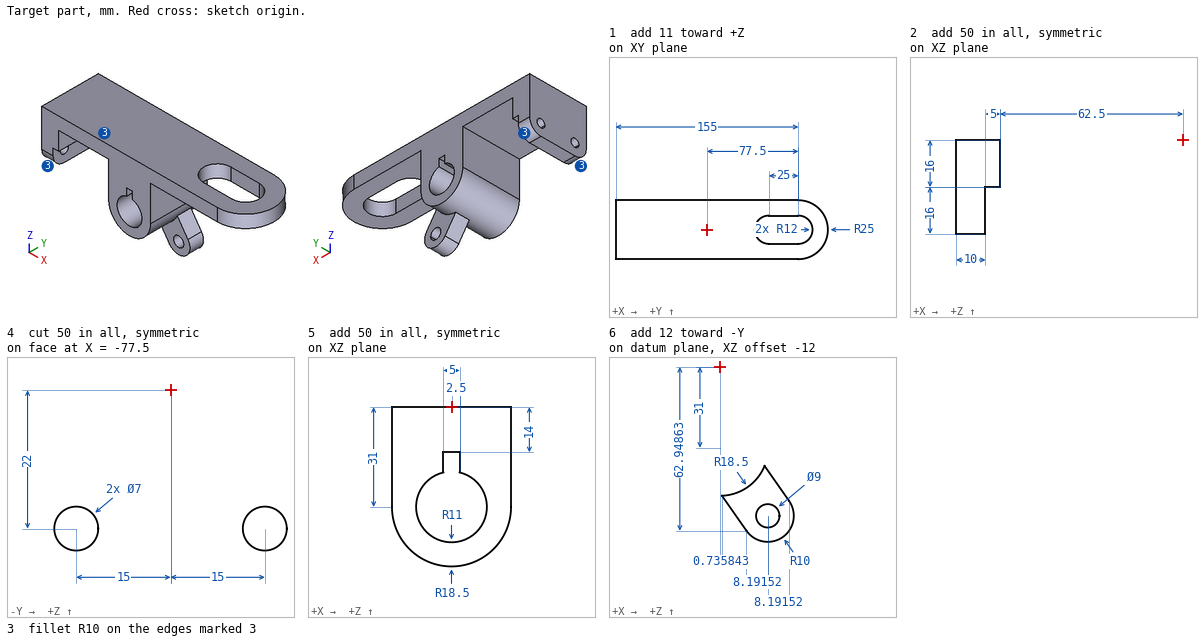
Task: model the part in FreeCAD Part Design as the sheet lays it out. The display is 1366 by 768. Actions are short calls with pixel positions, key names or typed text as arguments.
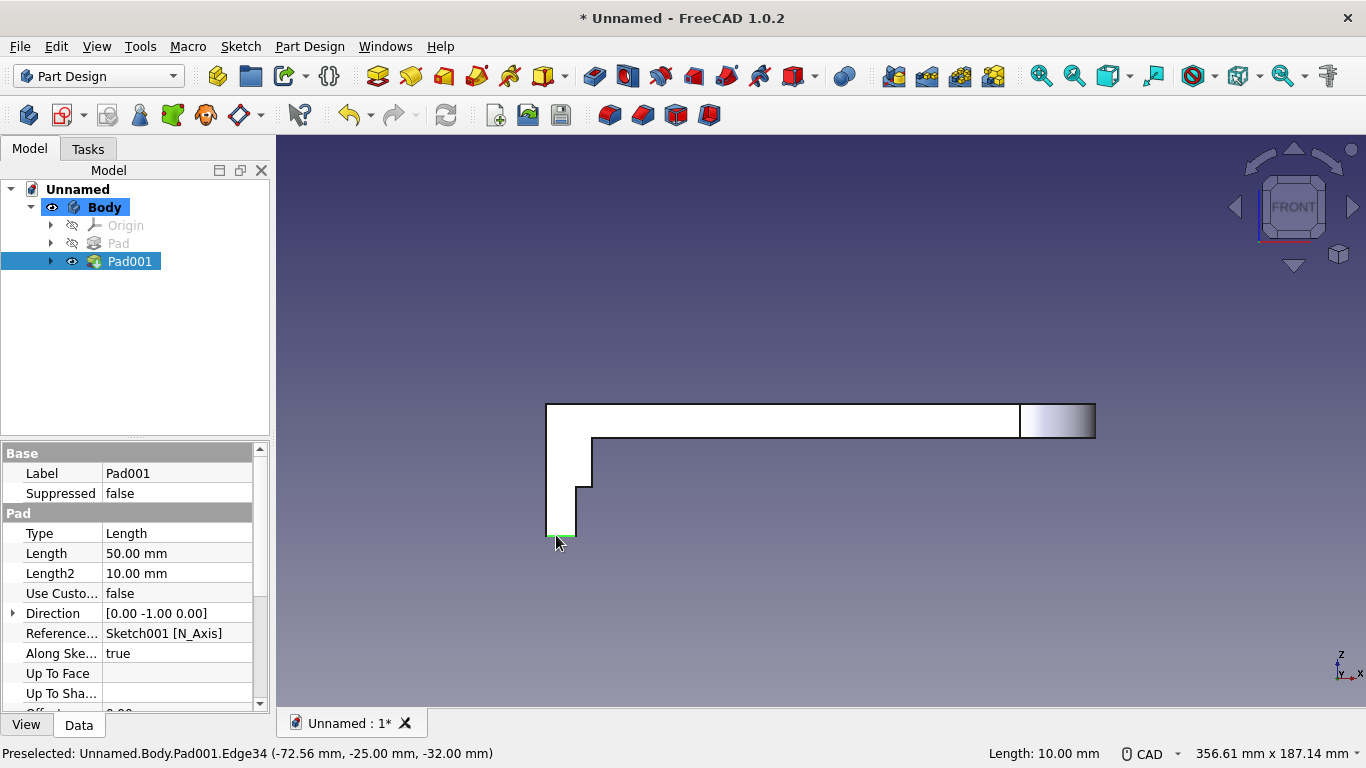
key(3)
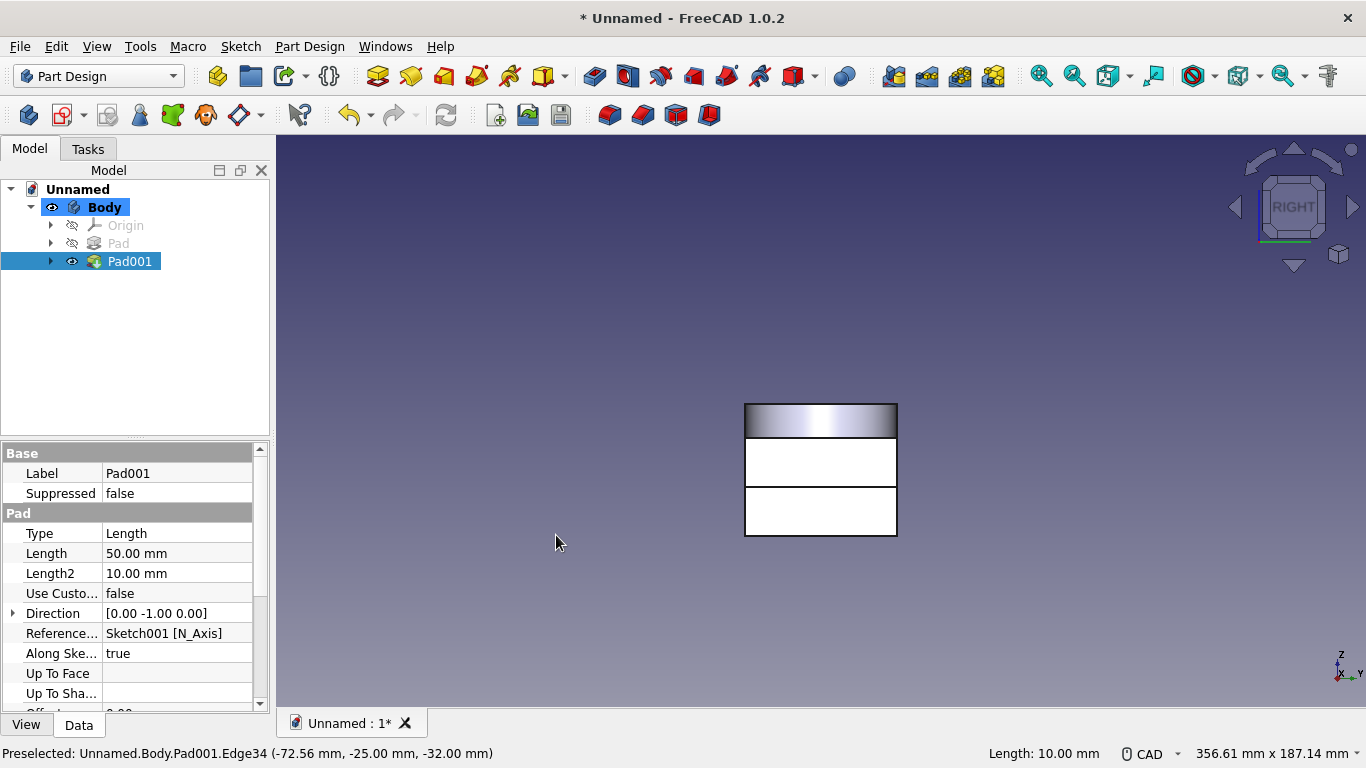
key(v)
key(f)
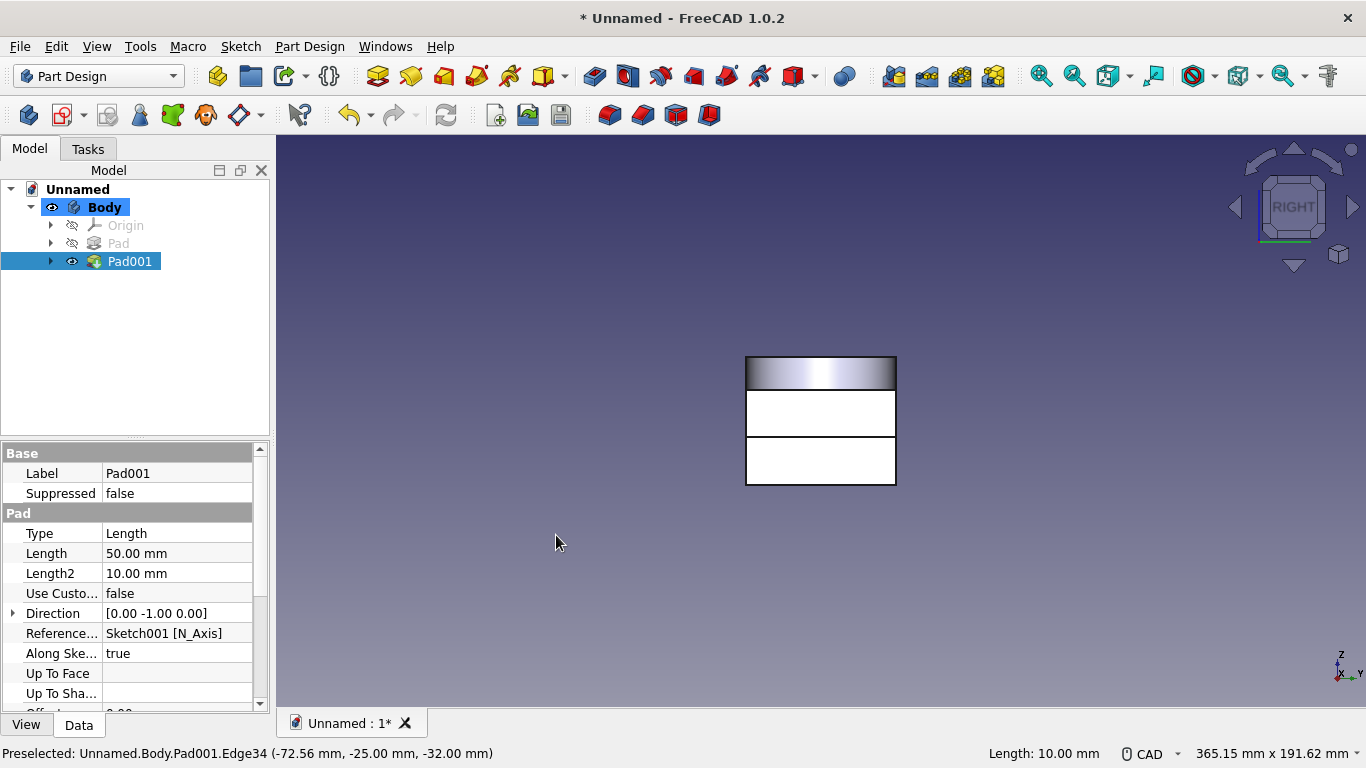
key(5)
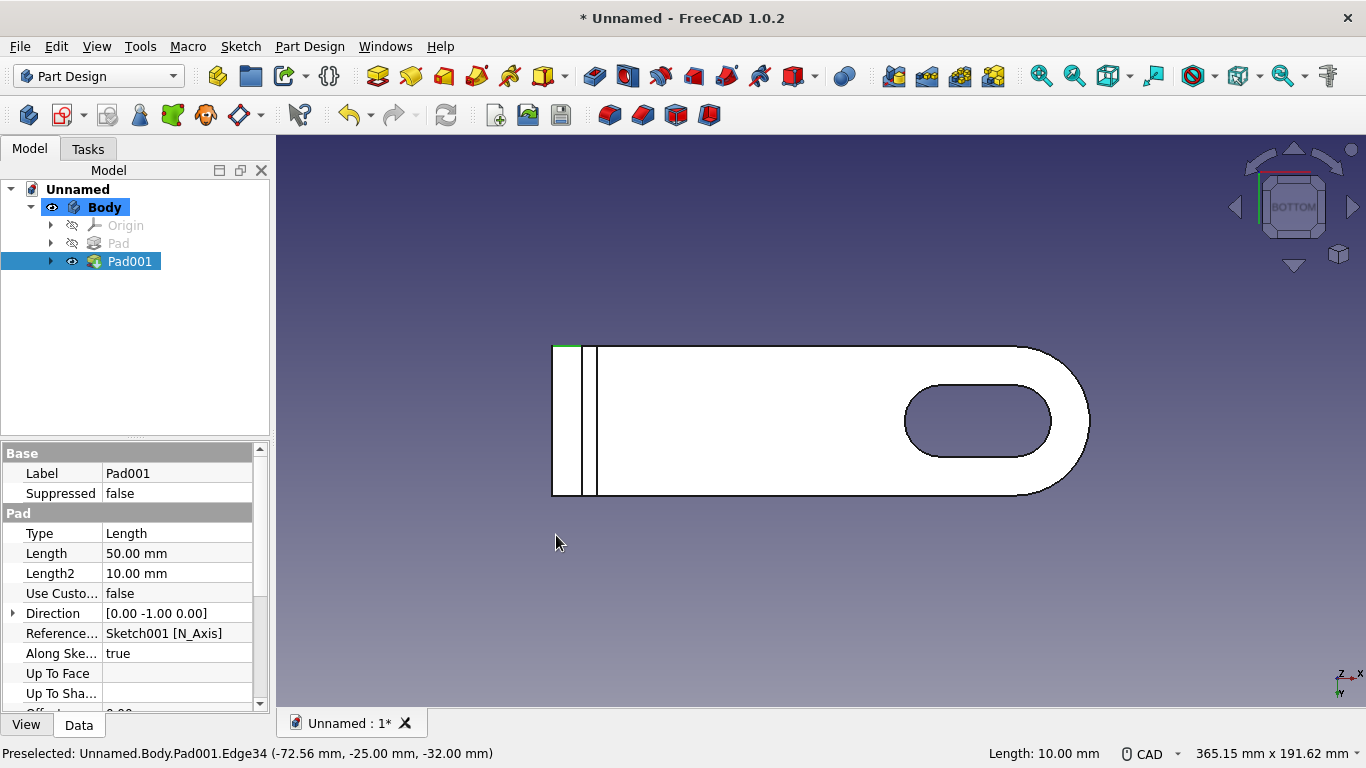
click(567, 495, ctrl)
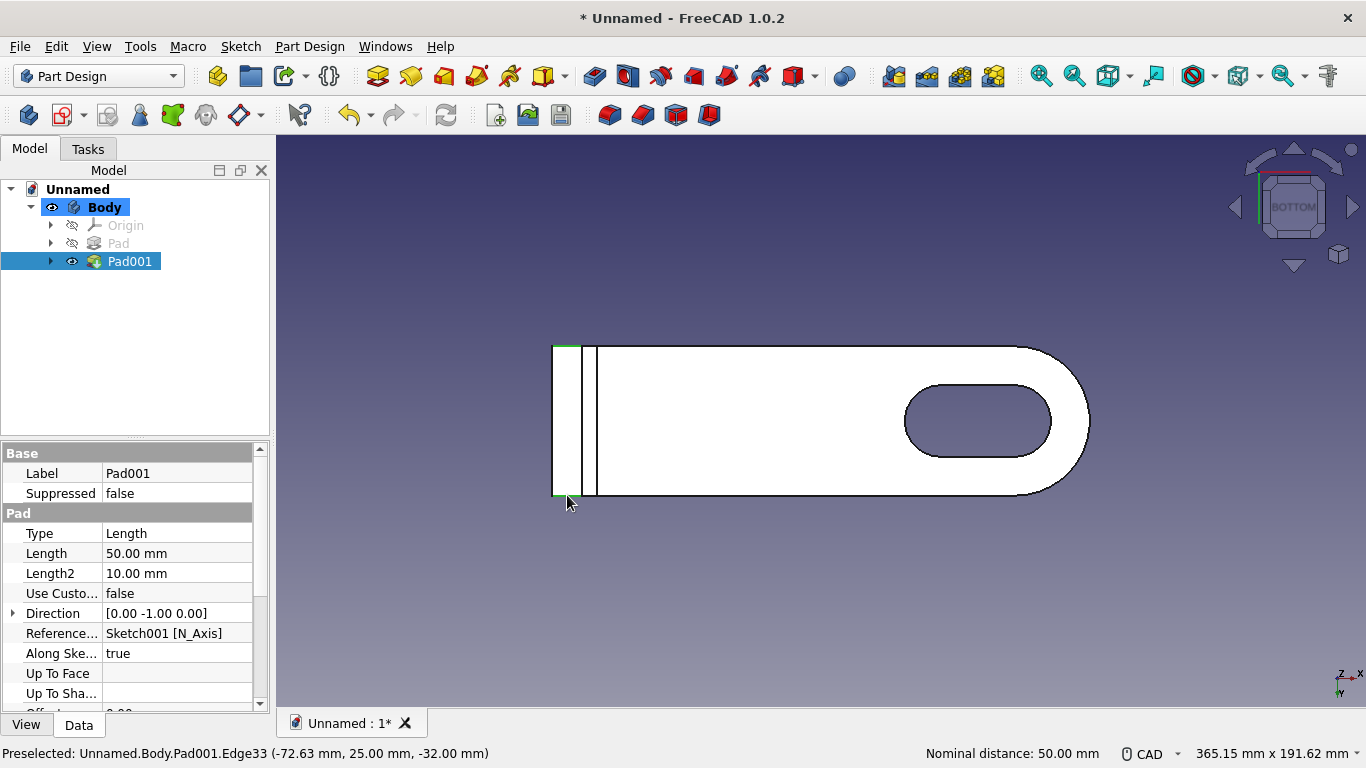
click(610, 116)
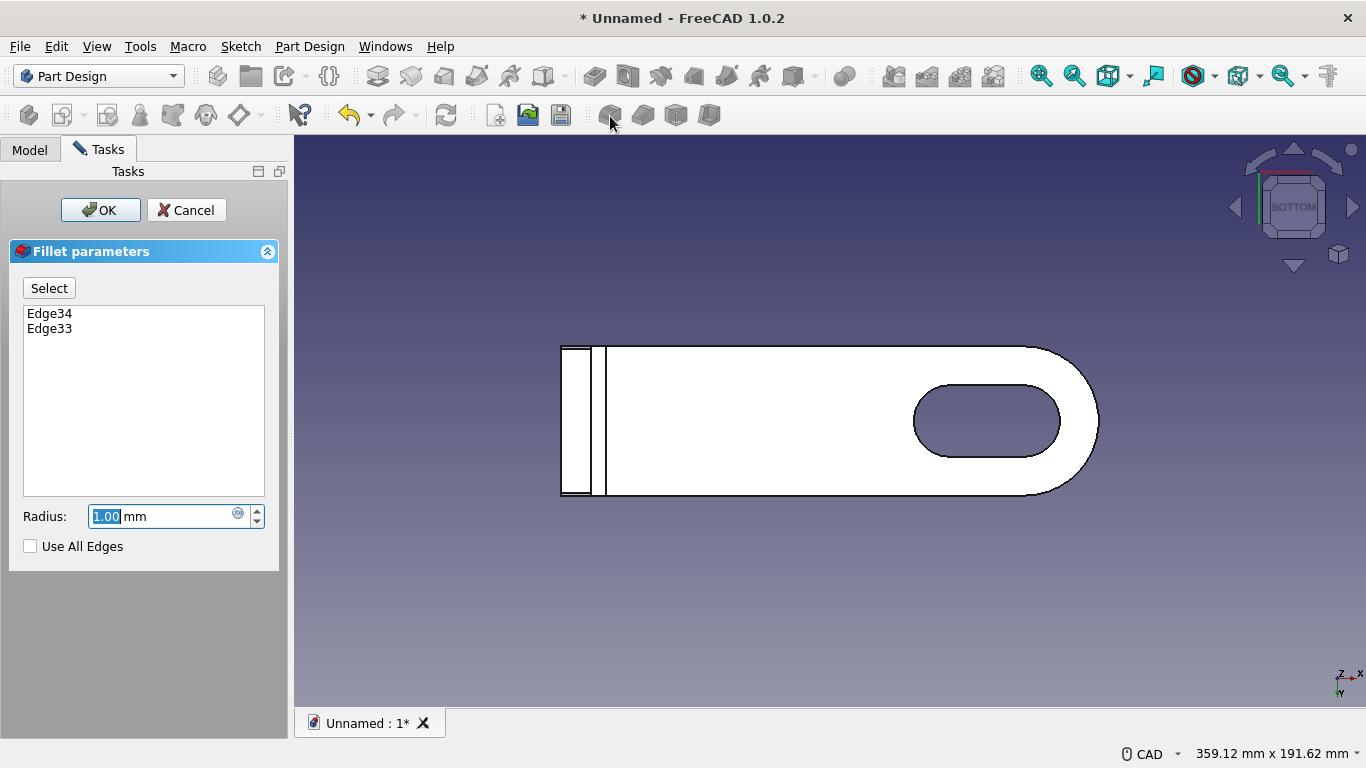
text(10)
key(Tab)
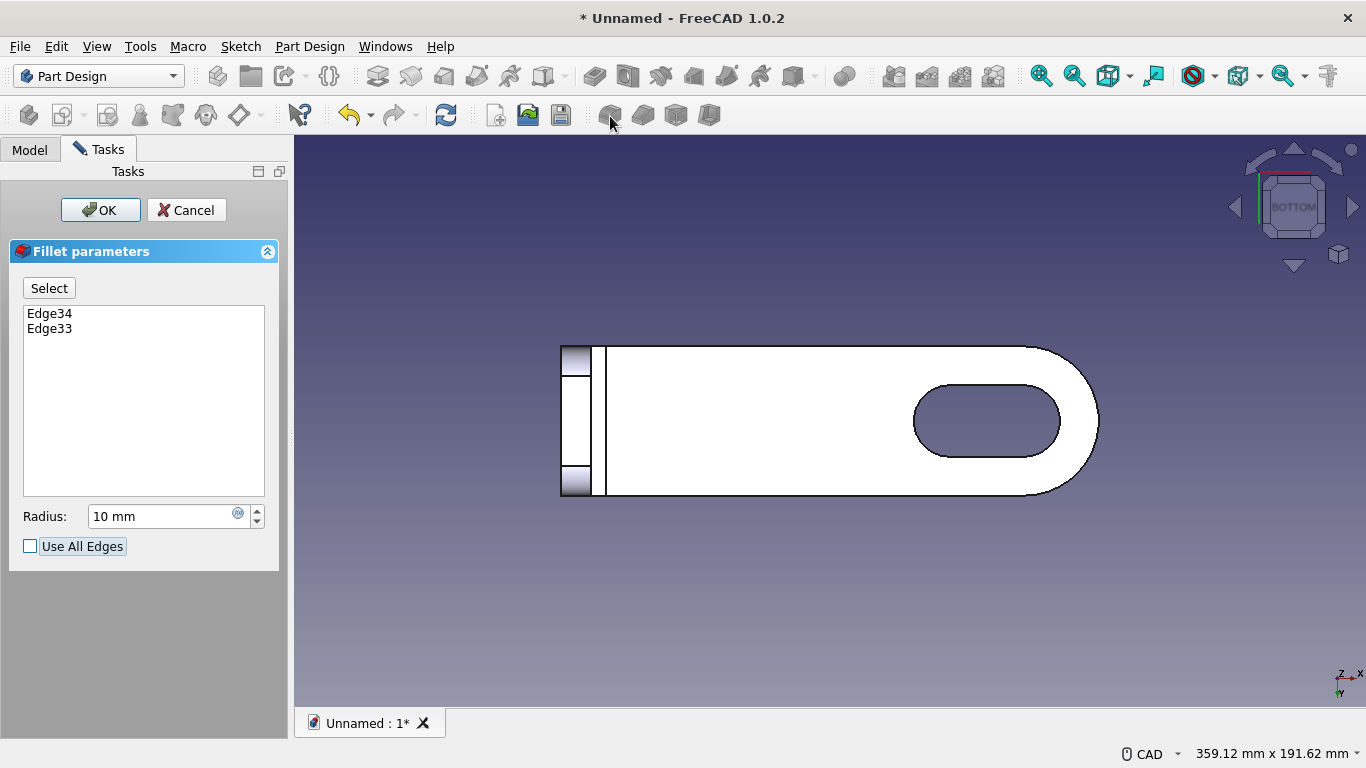
click(101, 210)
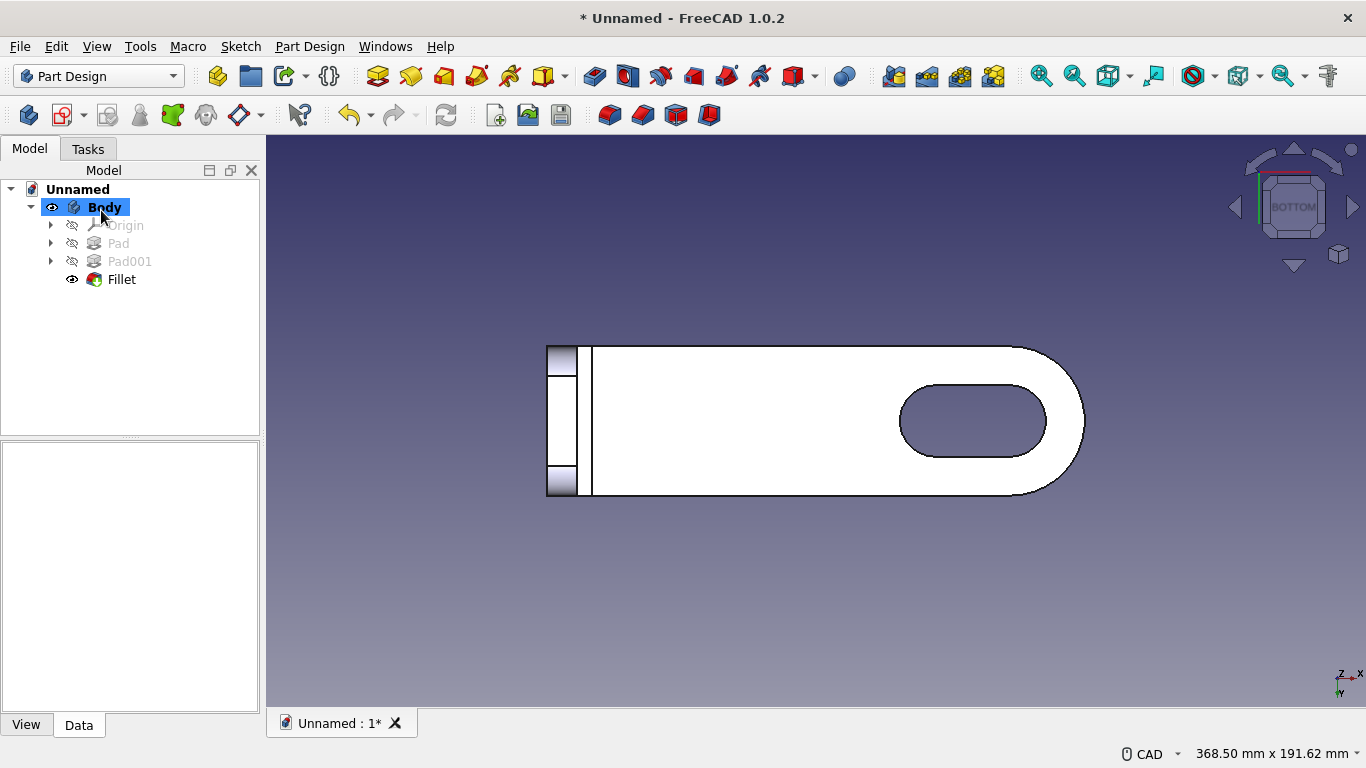
key(6)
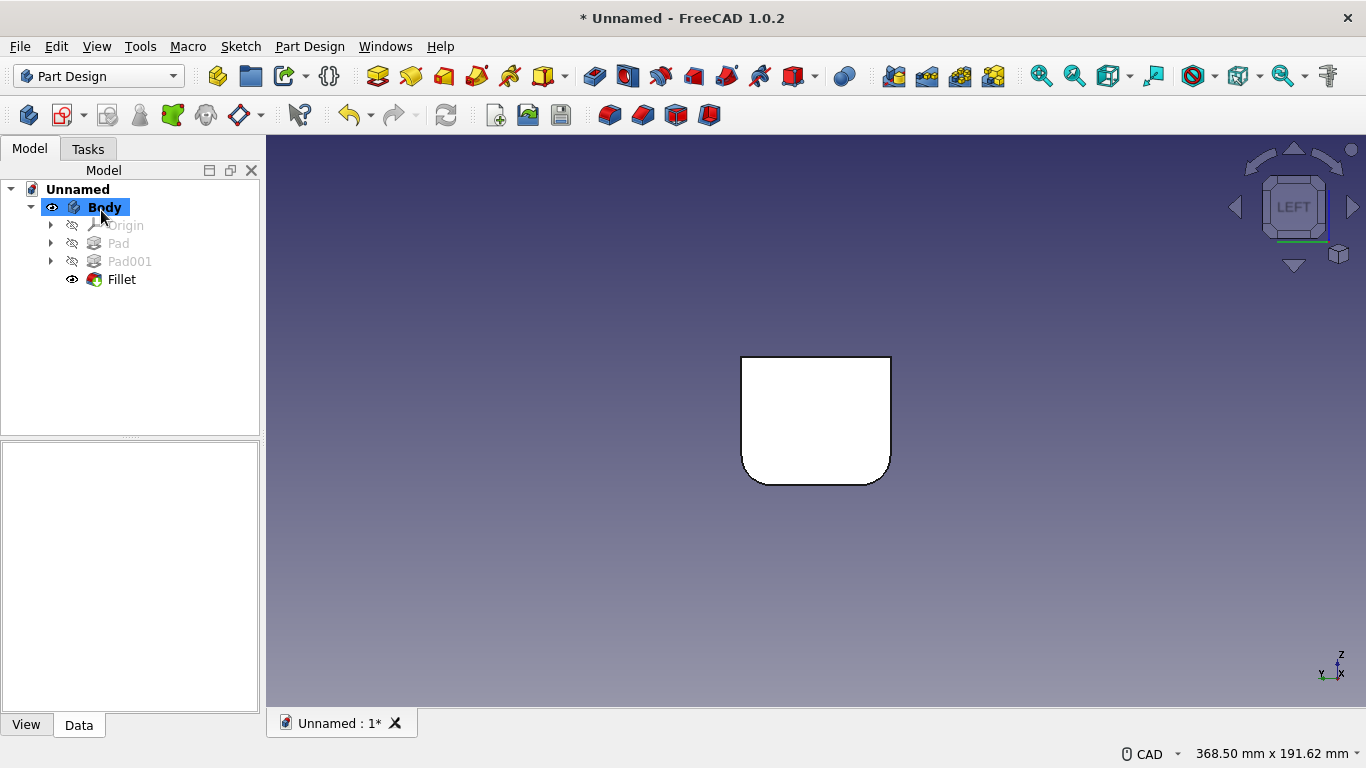
click(1042, 76)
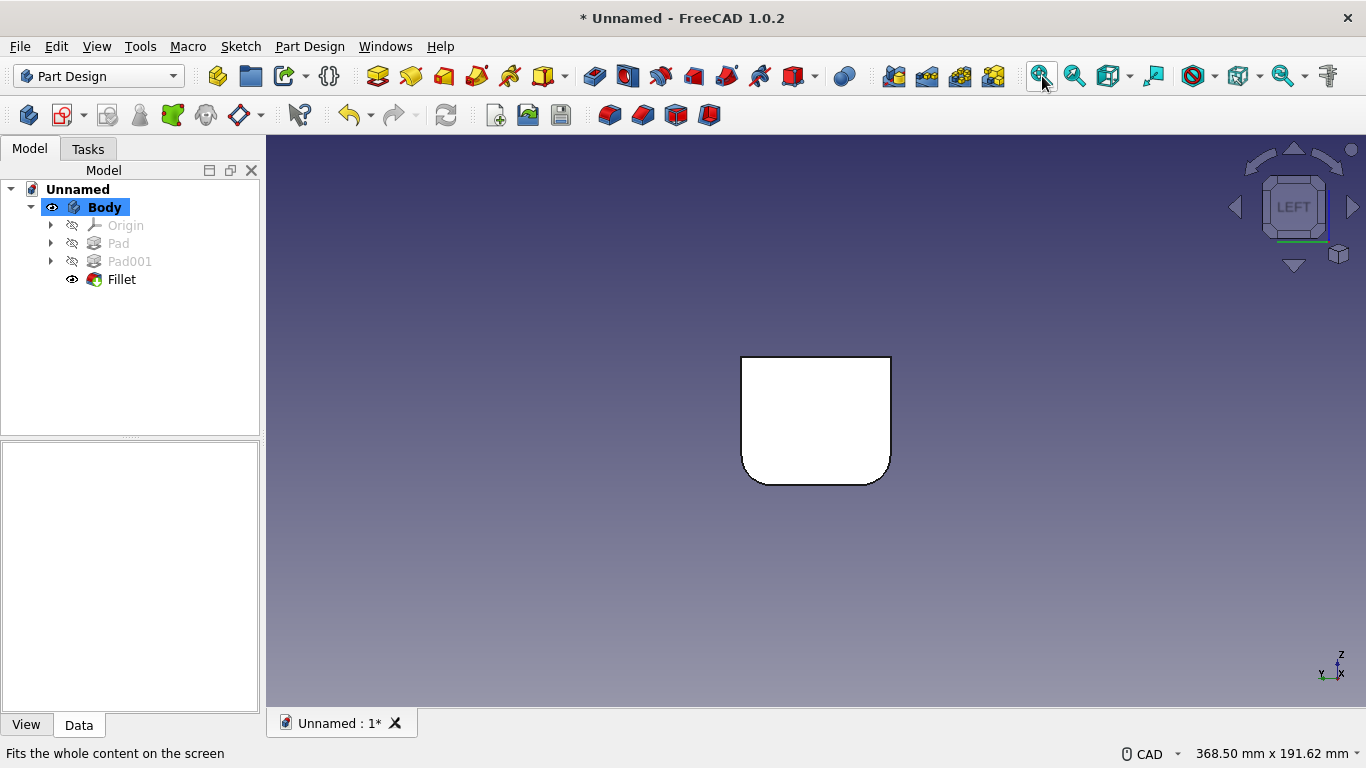
click(816, 420)